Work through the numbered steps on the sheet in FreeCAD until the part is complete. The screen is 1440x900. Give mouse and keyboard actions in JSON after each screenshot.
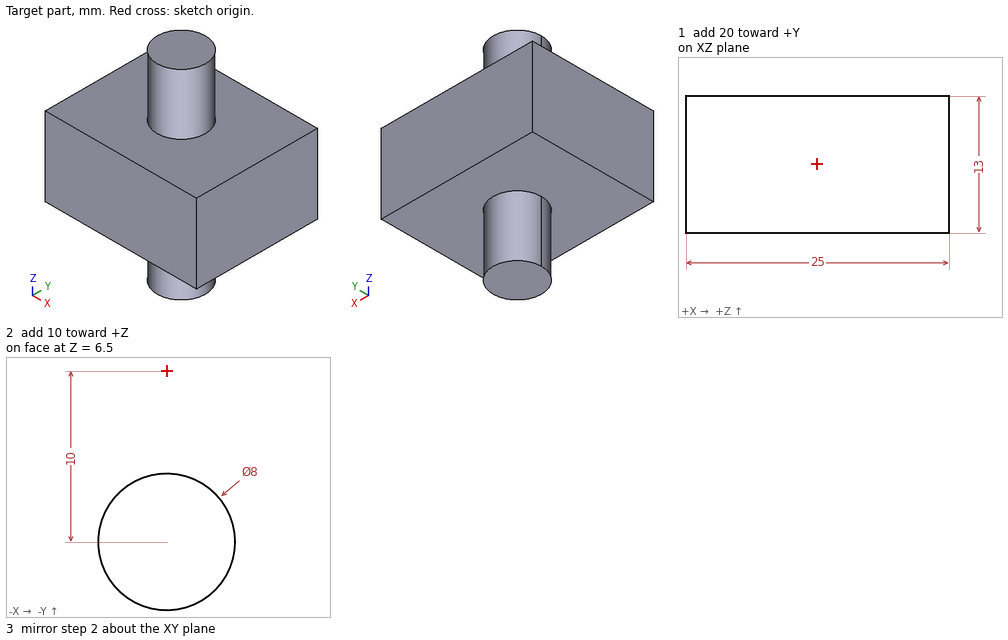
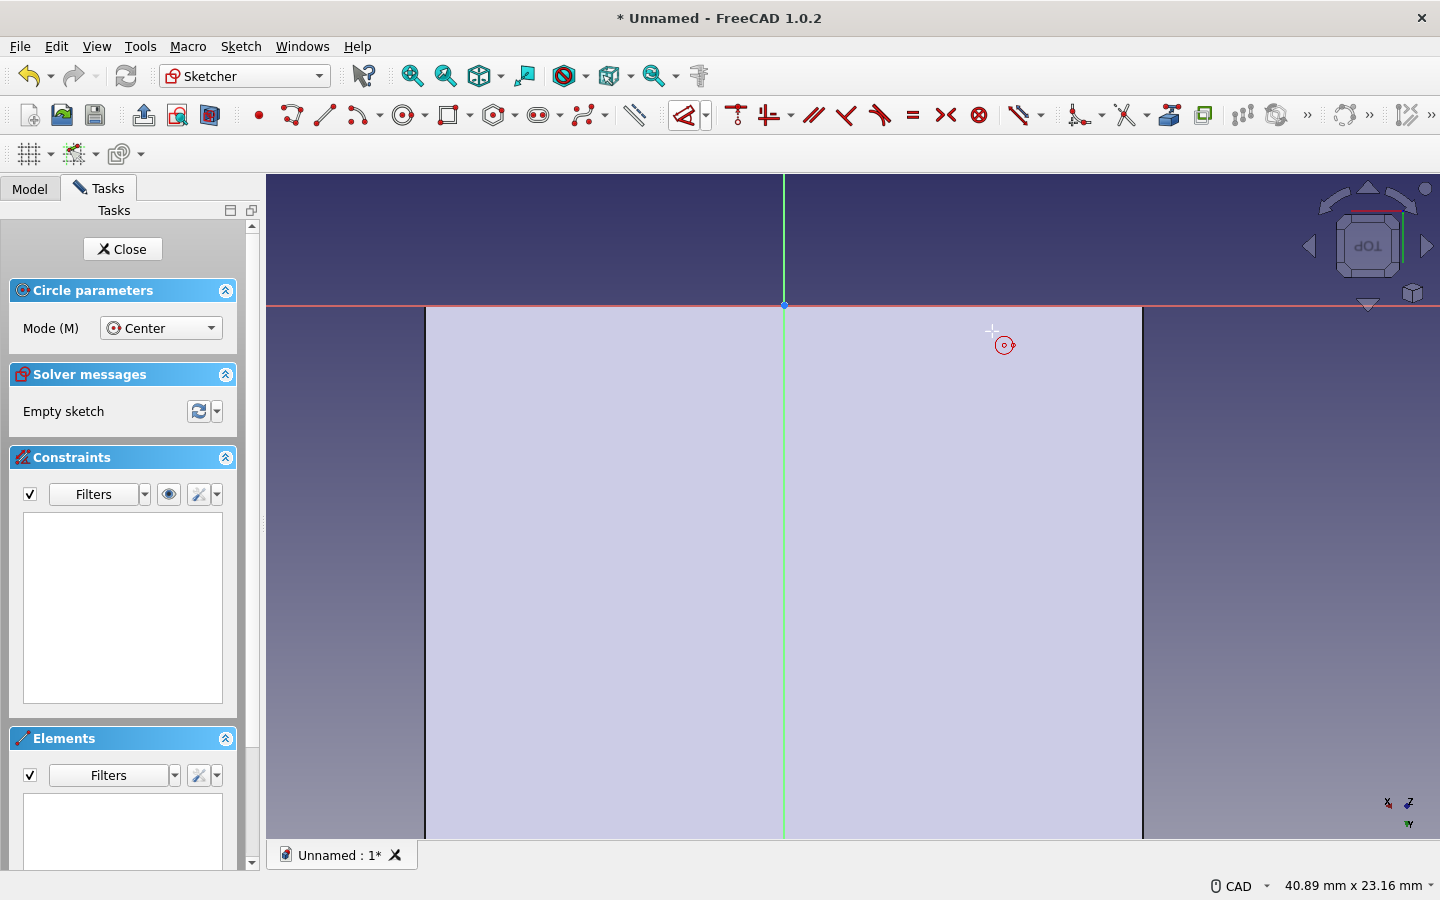
{"action": "left_click", "coordinate": [784, 593]}
{"action": "left_click", "coordinate": [866, 511]}
{"action": "key", "text": "Escape"}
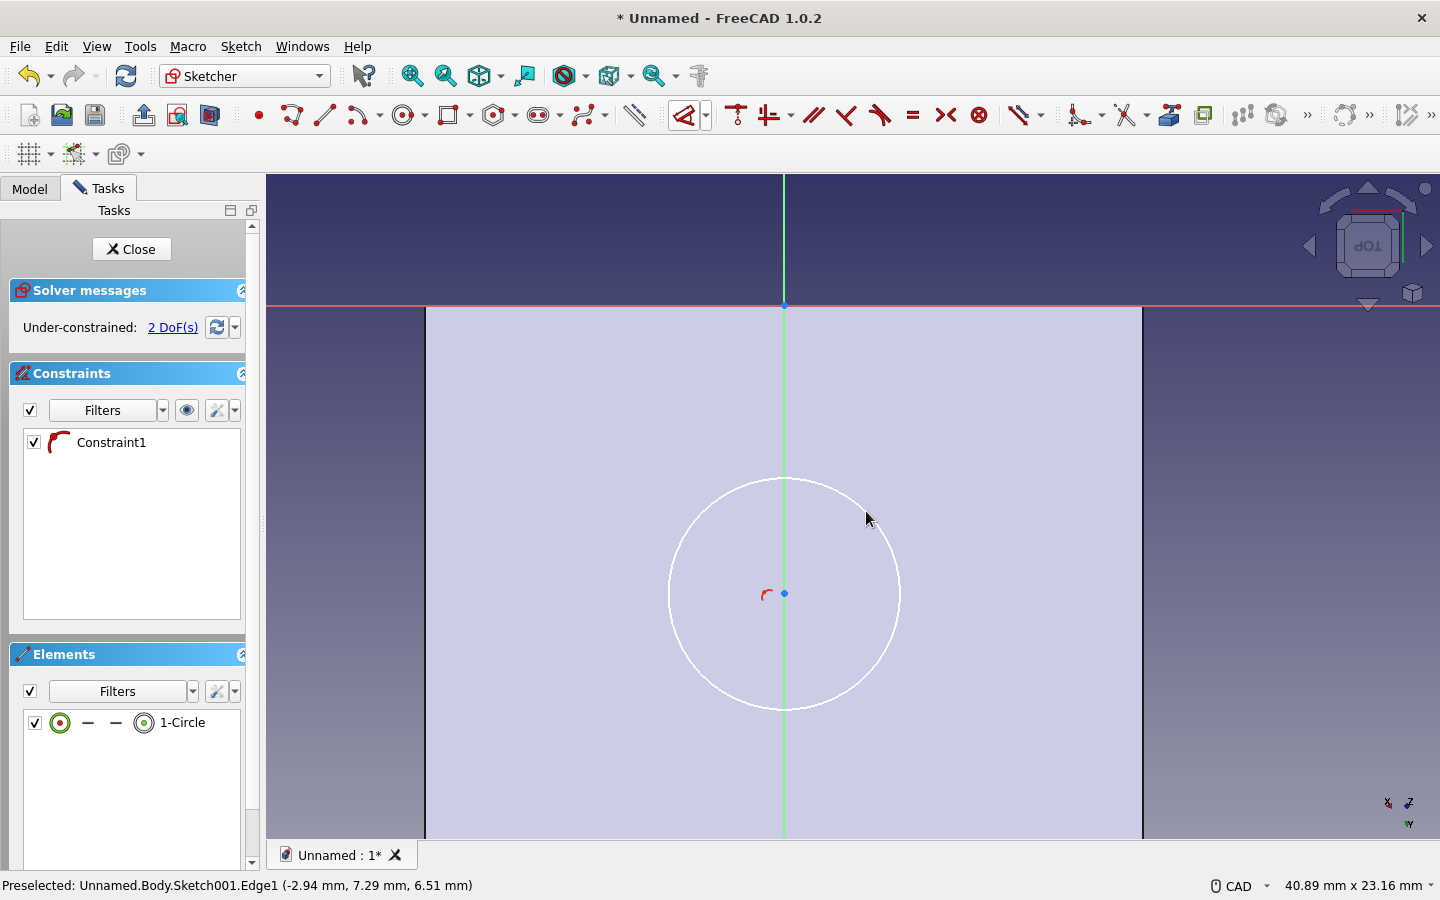
{"action": "left_click", "coordinate": [866, 512]}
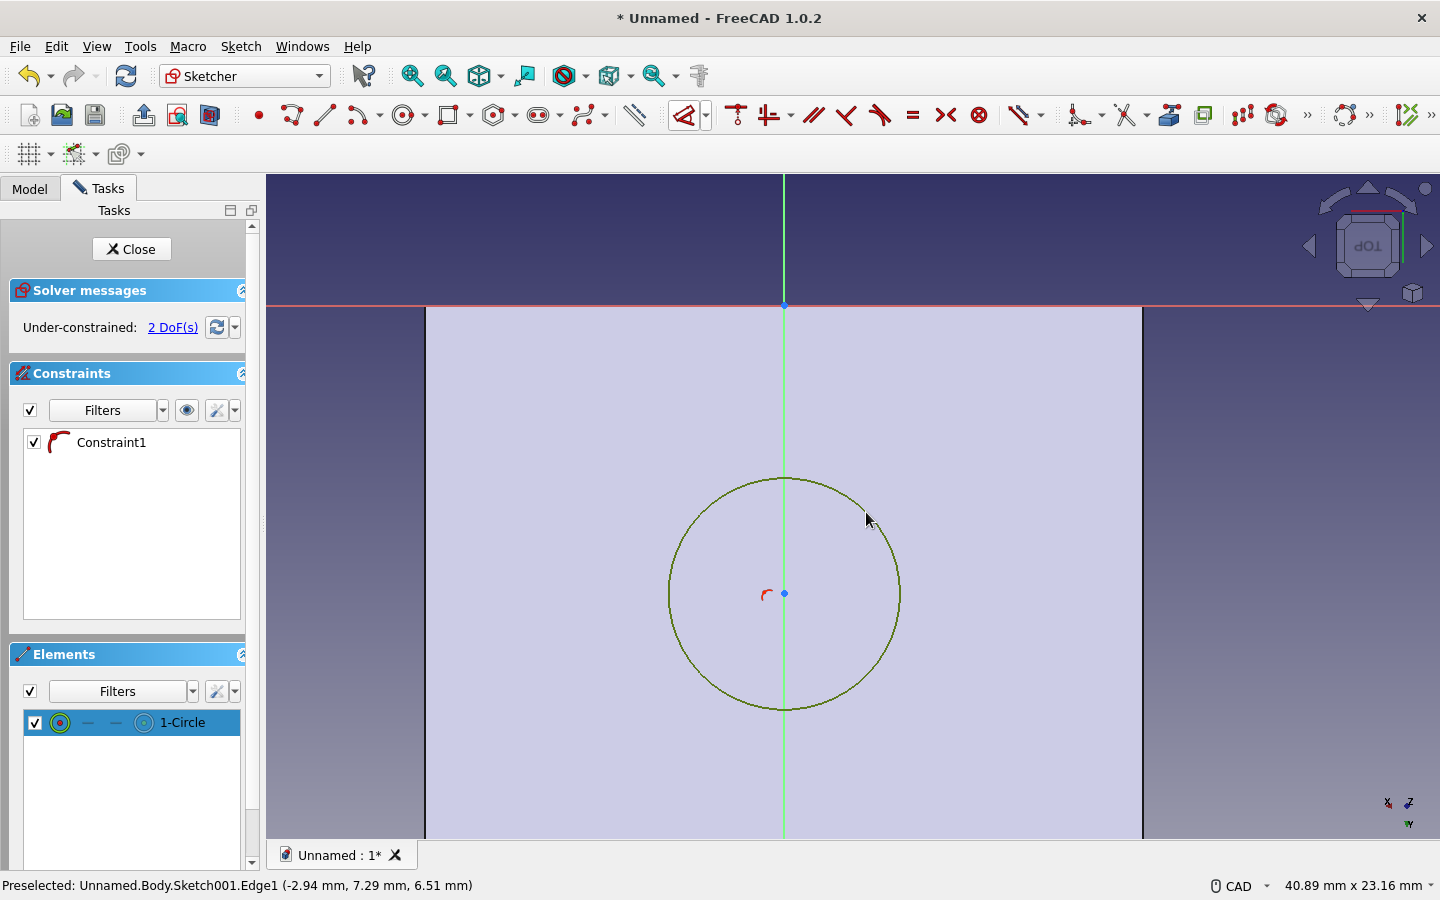
{"action": "left_click", "coordinate": [706, 116]}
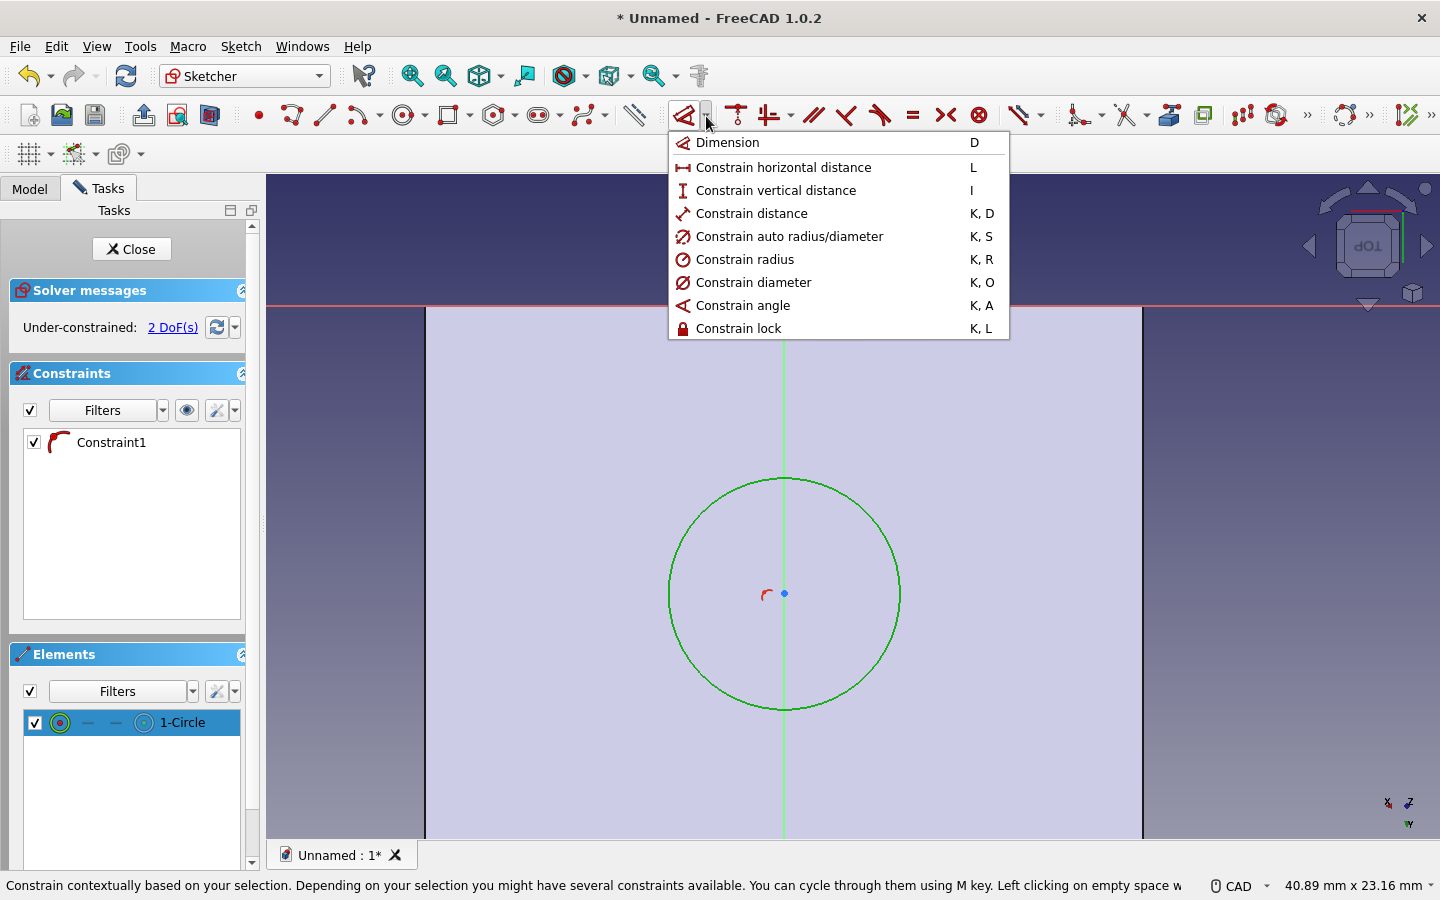
{"action": "left_click", "coordinate": [839, 282]}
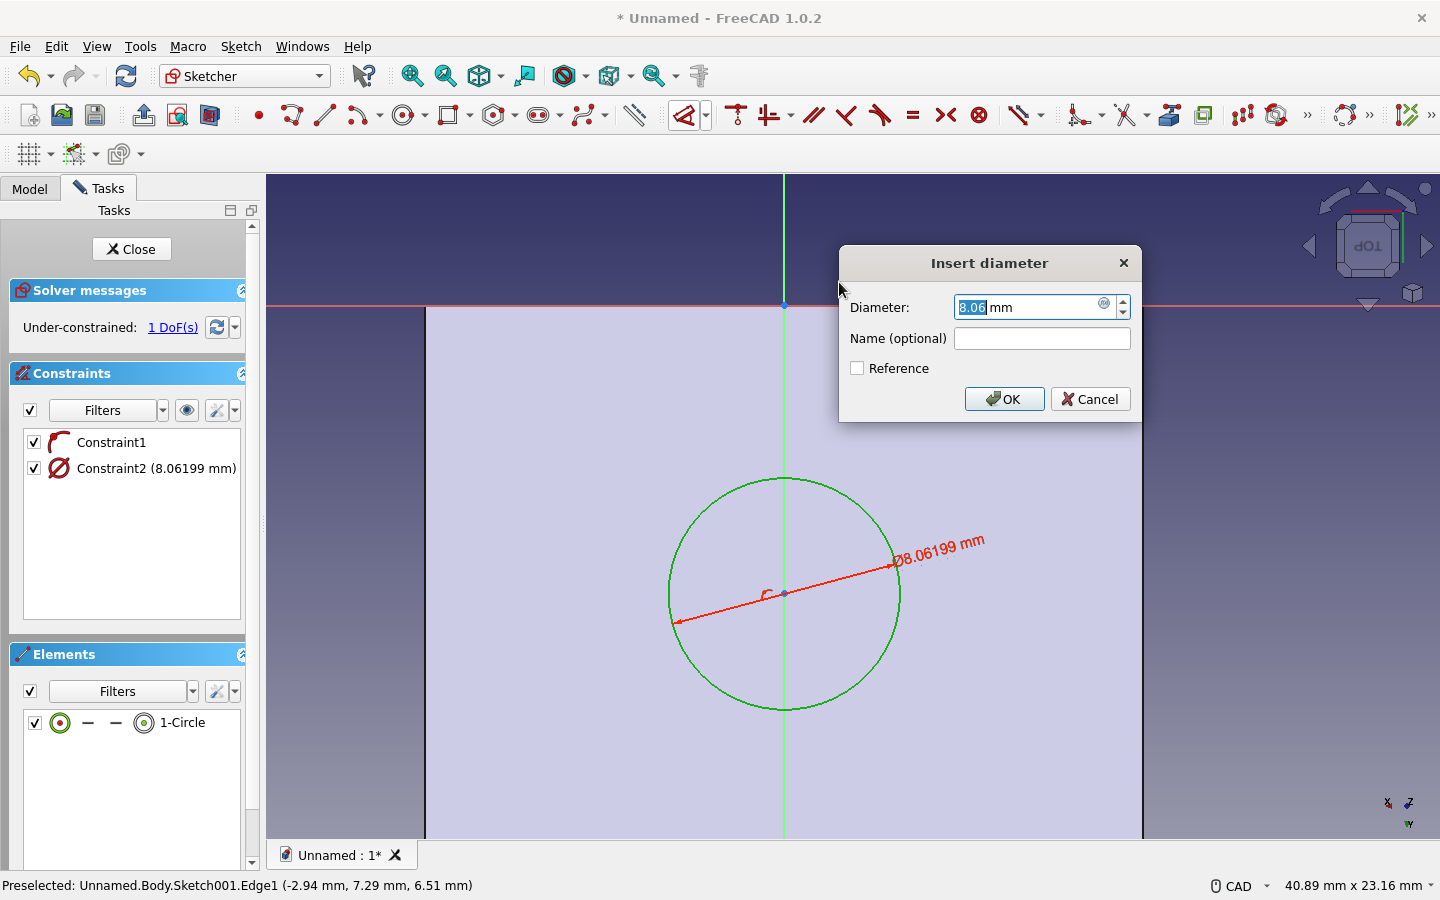
{"action": "type", "text": "8"}
{"action": "key", "text": "Return"}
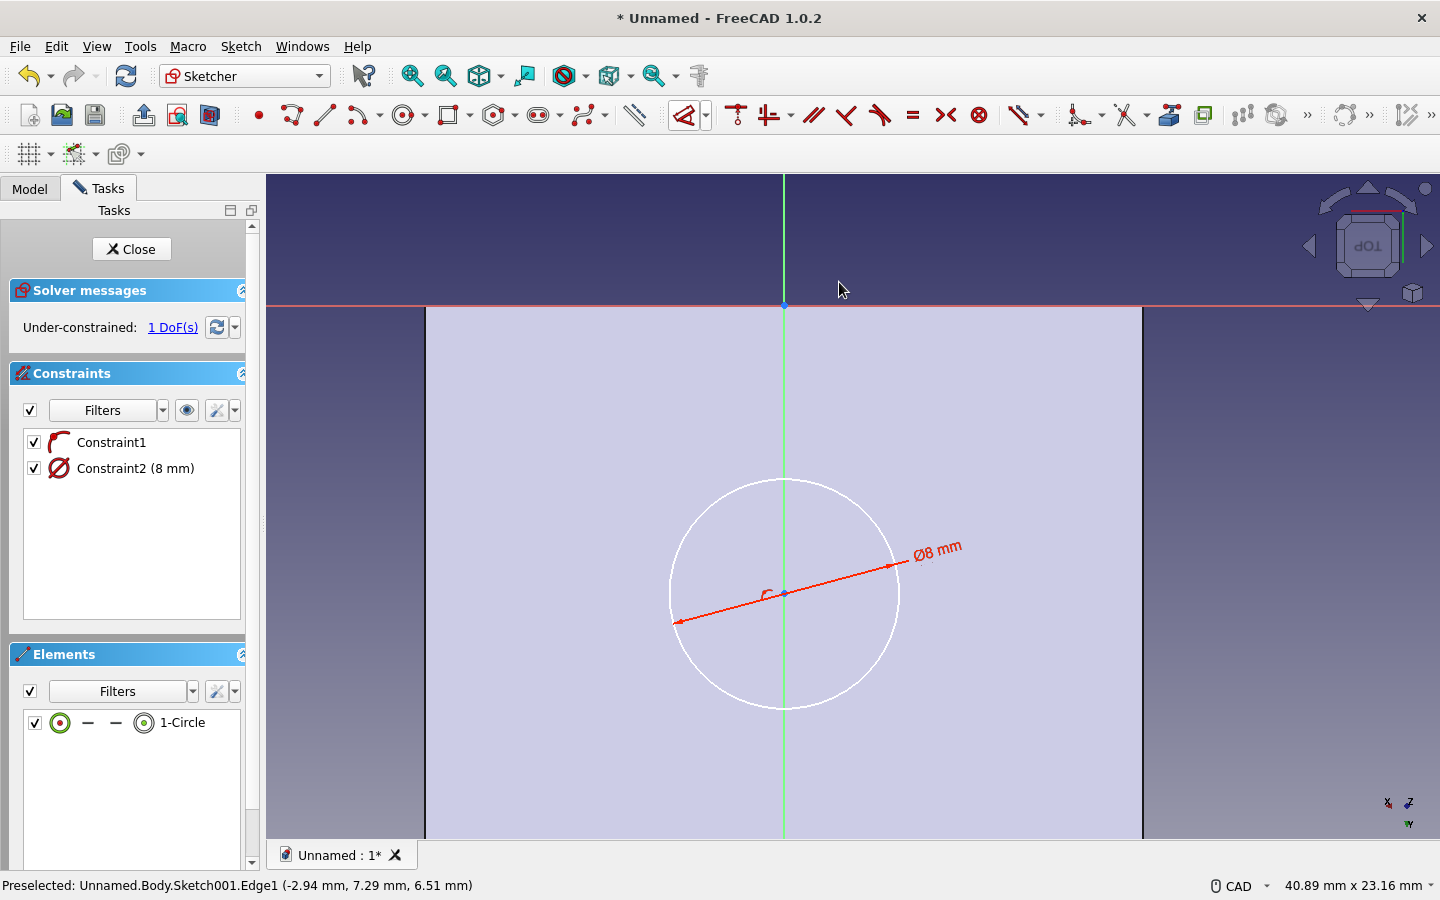
{"action": "left_click", "coordinate": [784, 594]}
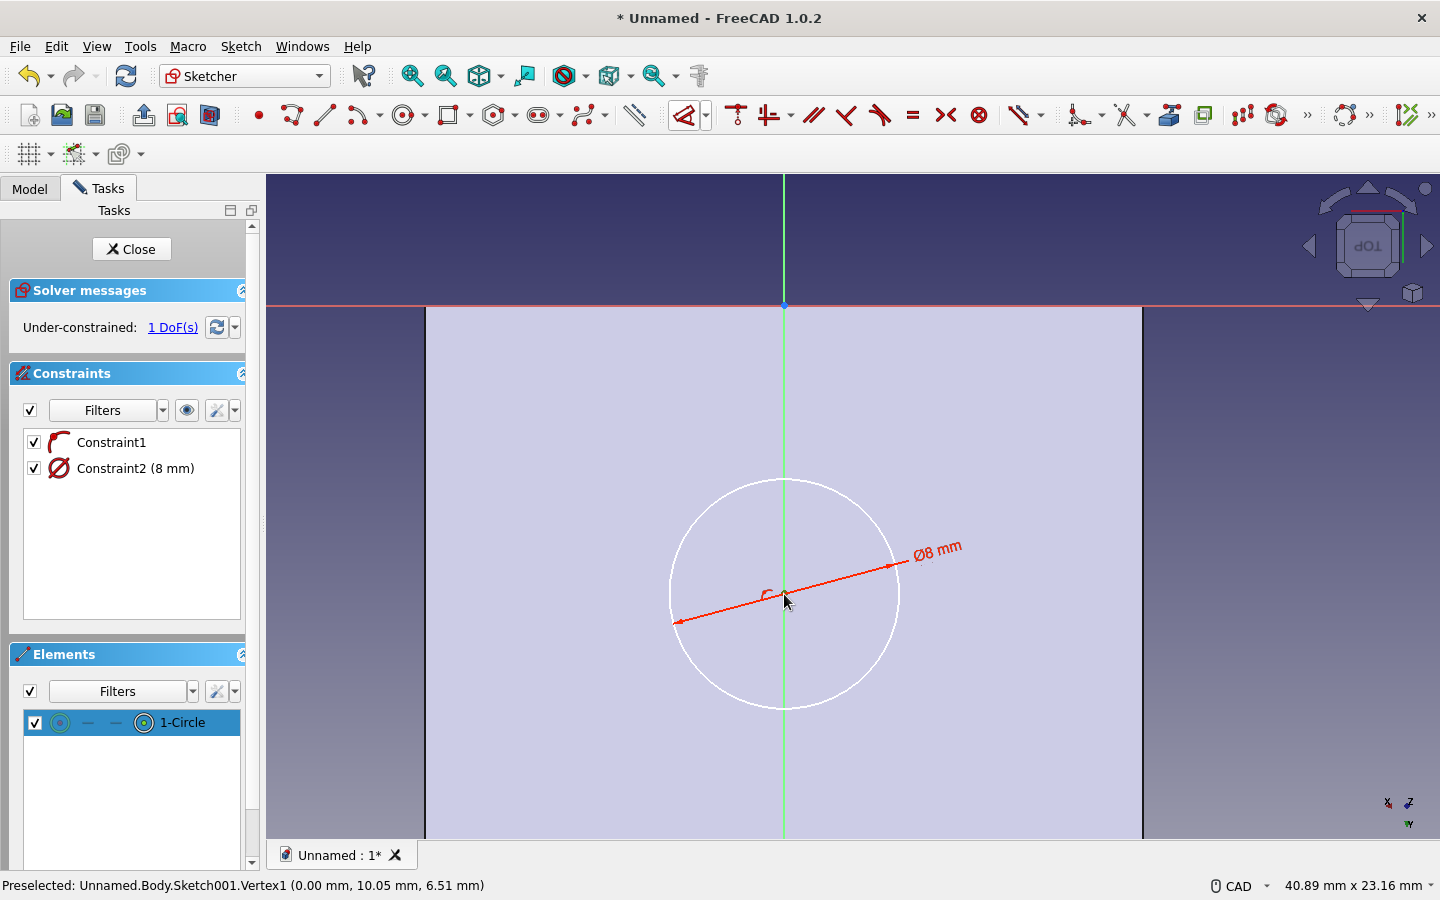
{"action": "key", "text": "i"}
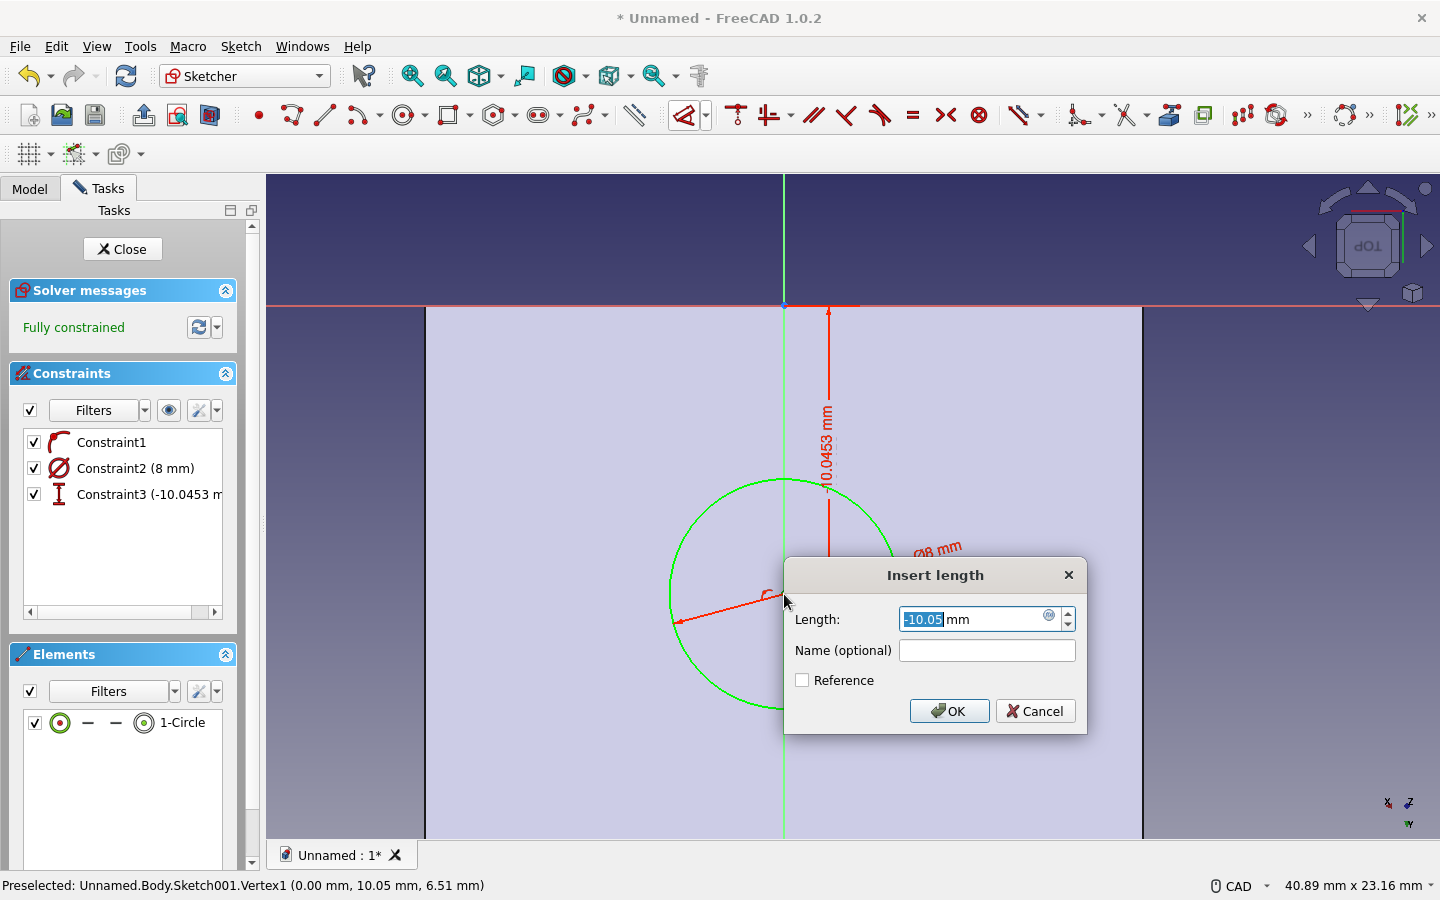
{"action": "type", "text": "-10"}
{"action": "key", "text": "Return"}